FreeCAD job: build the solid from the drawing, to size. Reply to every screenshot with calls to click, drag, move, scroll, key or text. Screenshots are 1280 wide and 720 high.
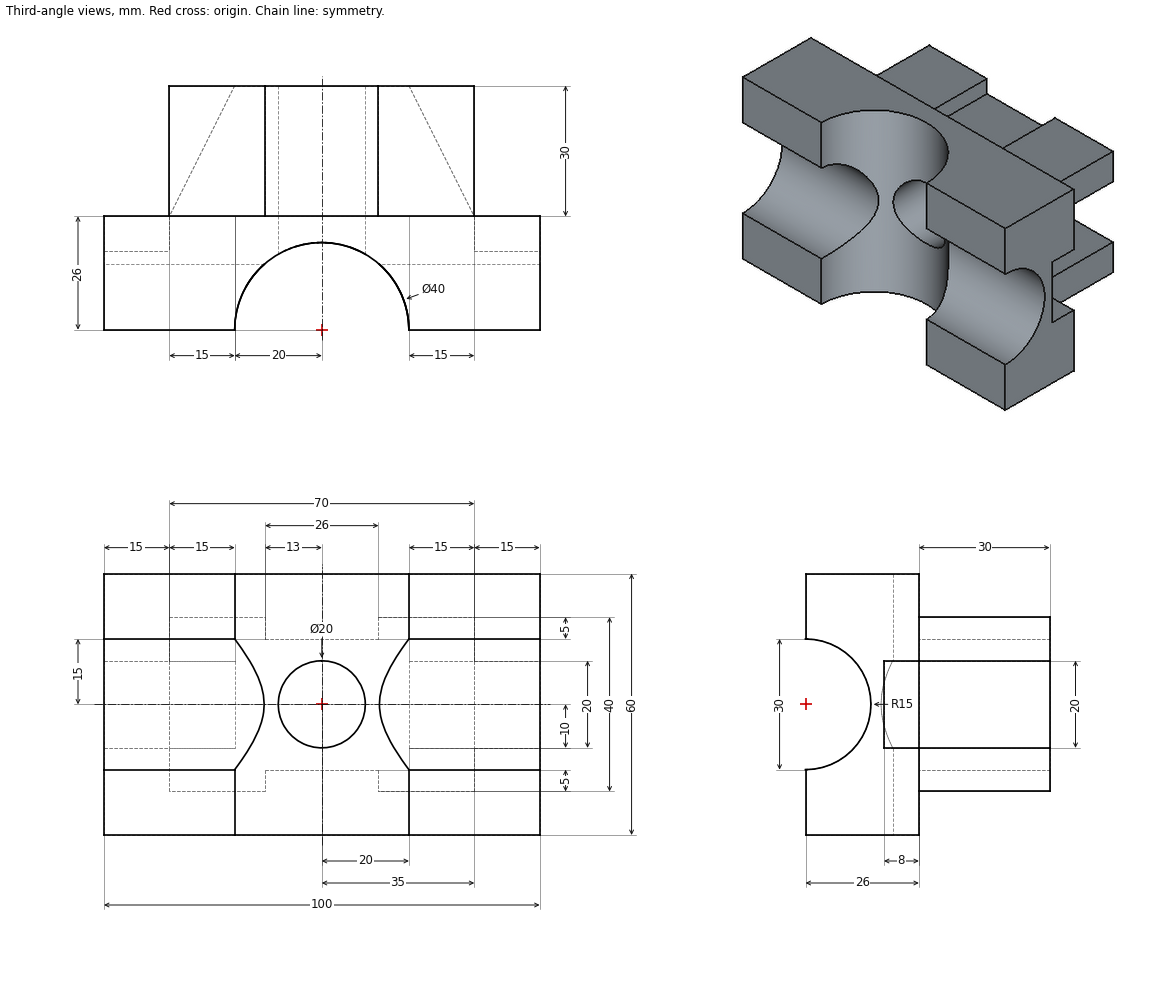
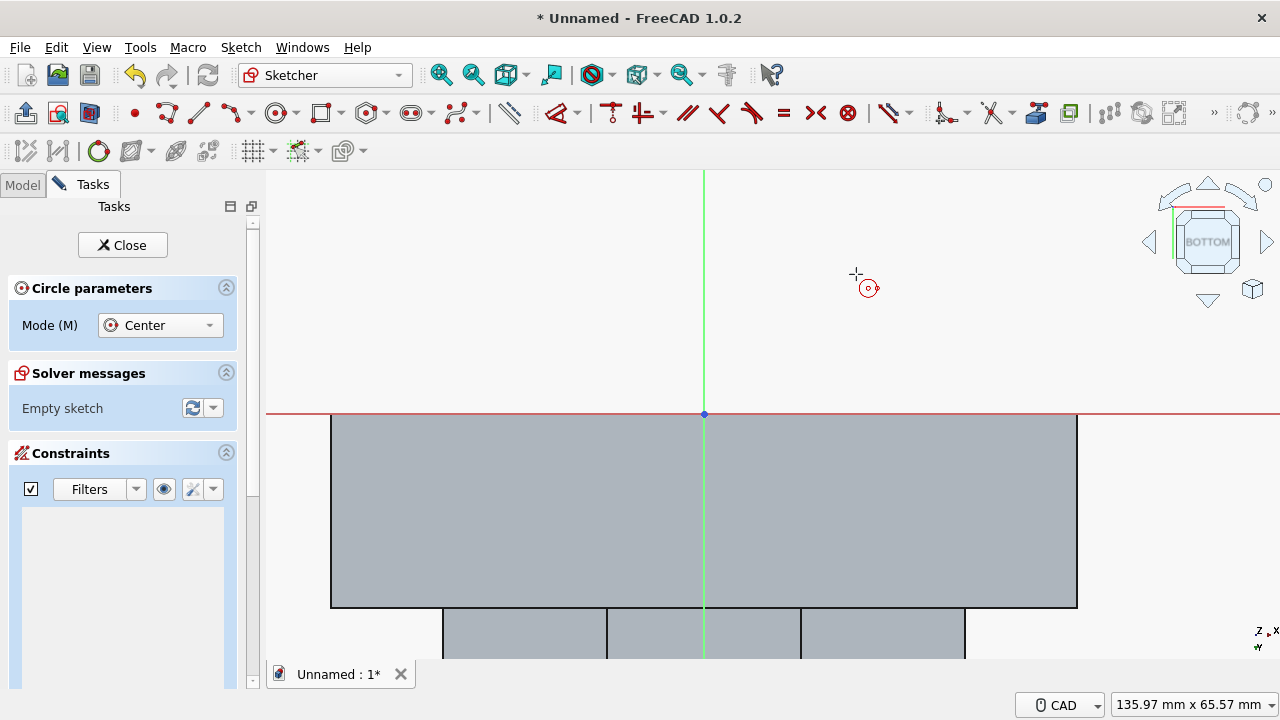
click(704, 414)
move(810, 309)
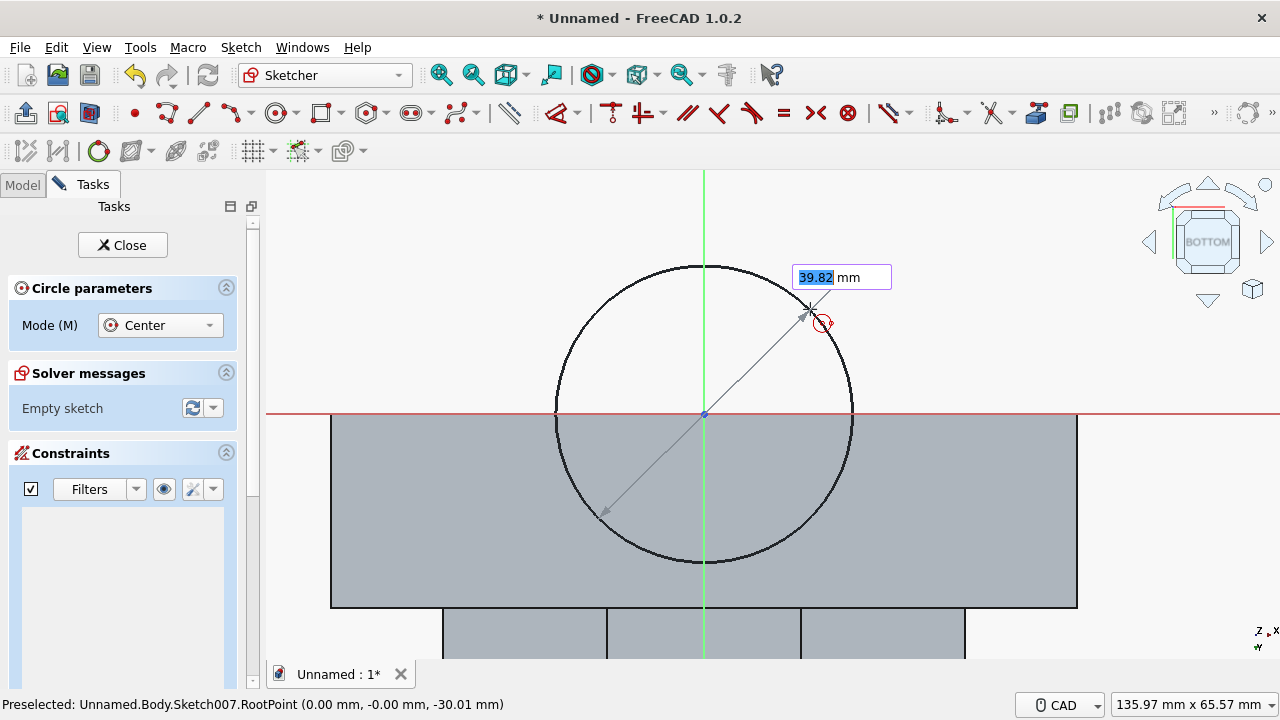
text(40)
key(Return)
key(Escape)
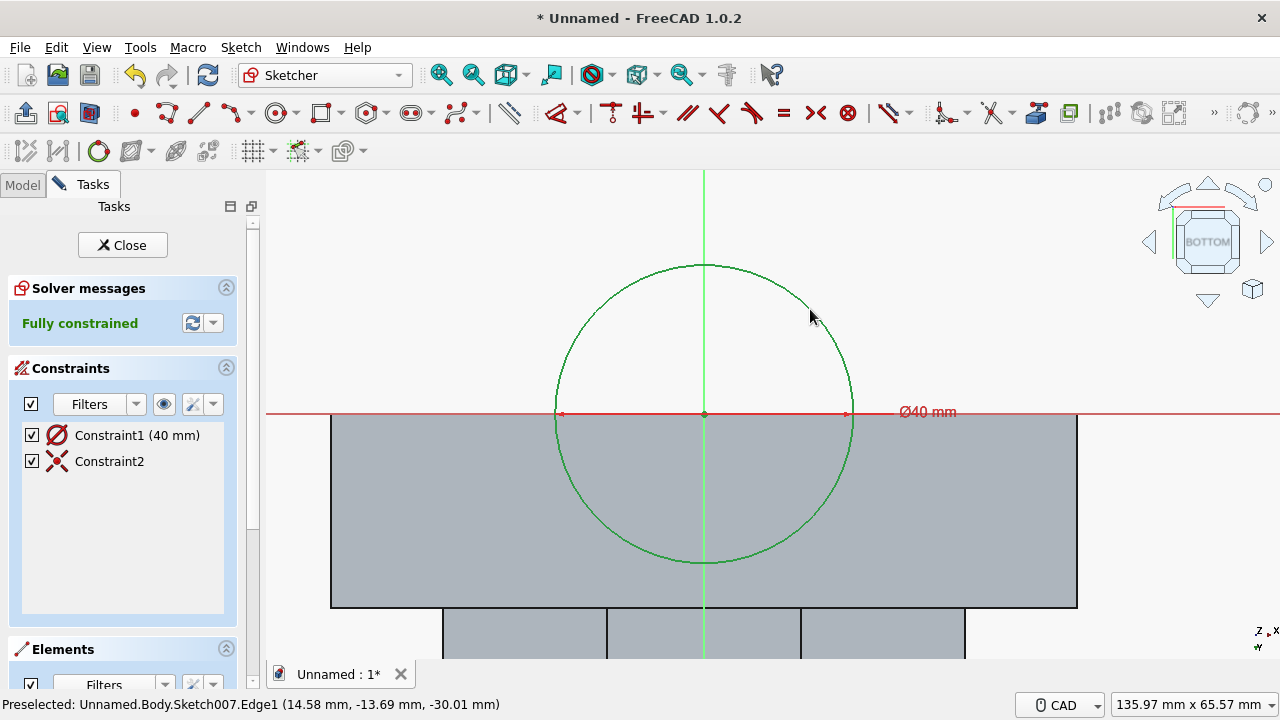
click(123, 245)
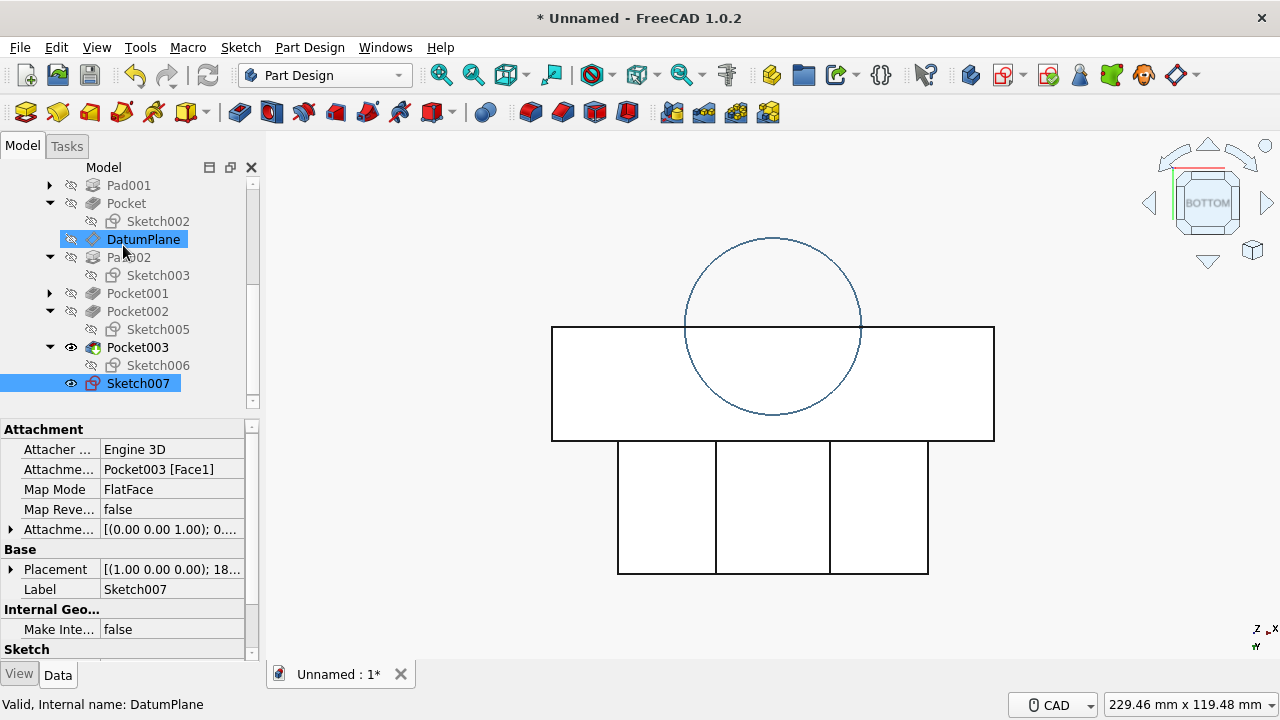
click(240, 112)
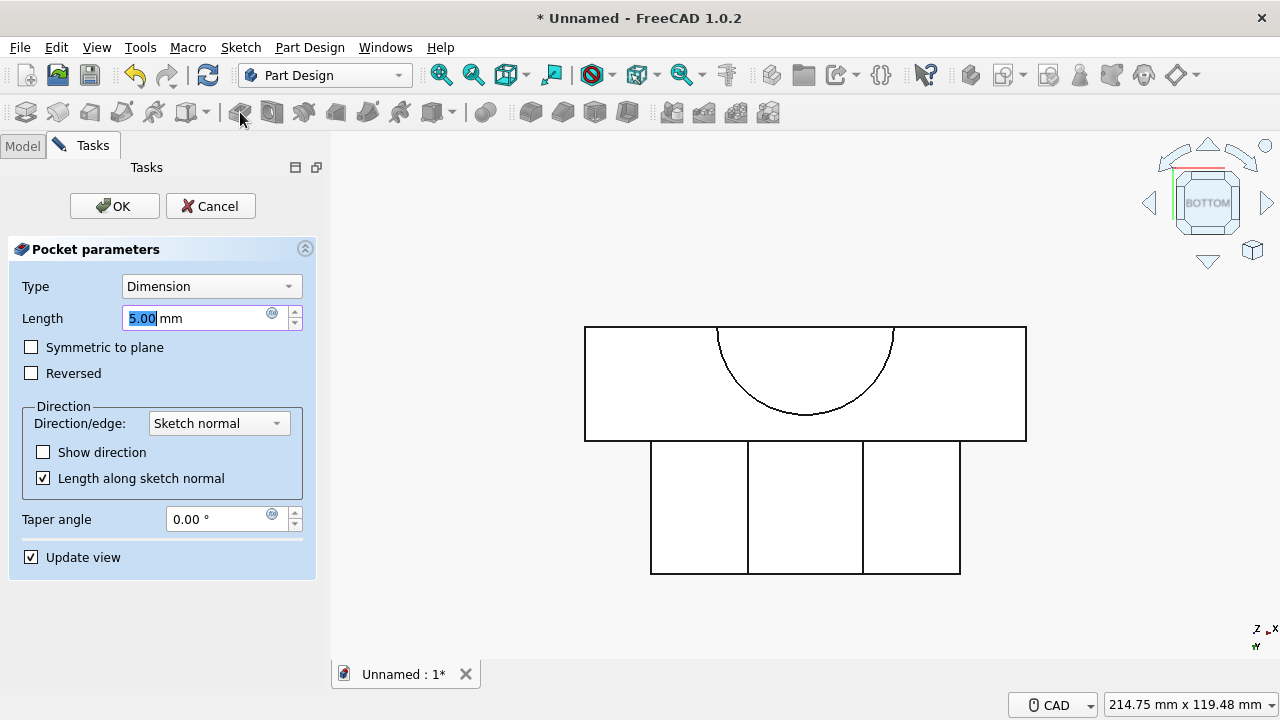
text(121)
key(Tab)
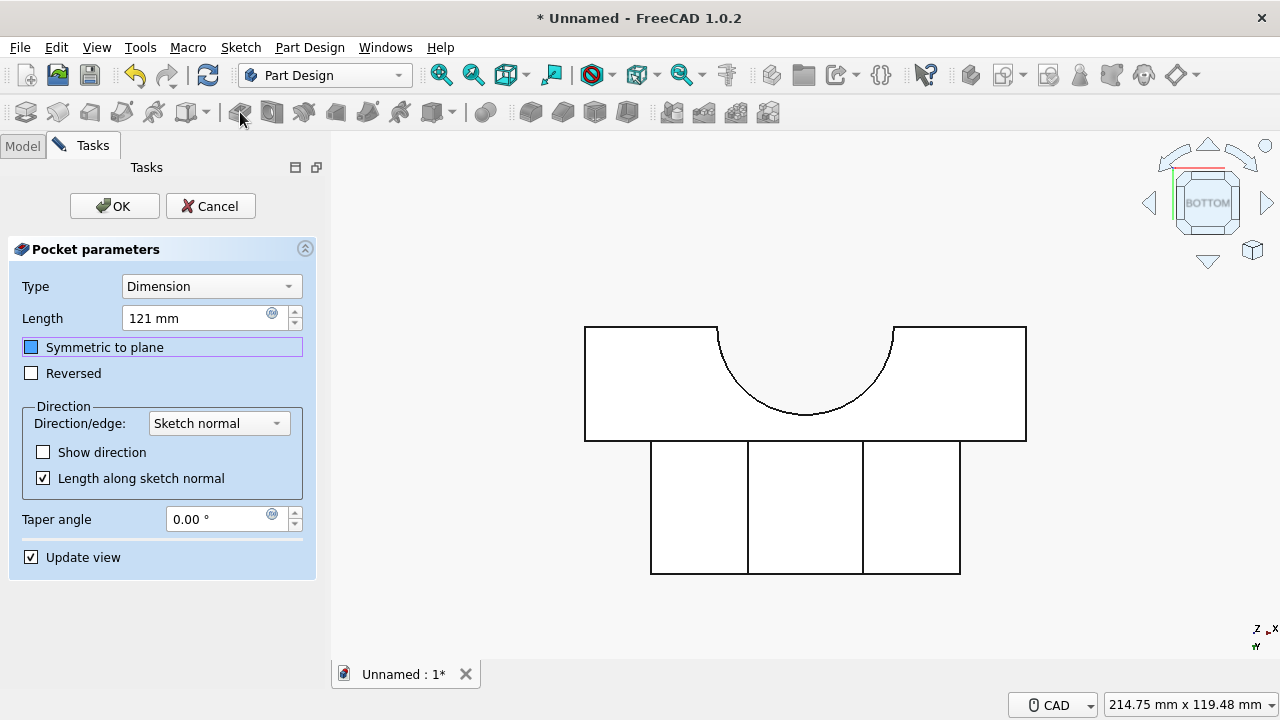
click(115, 206)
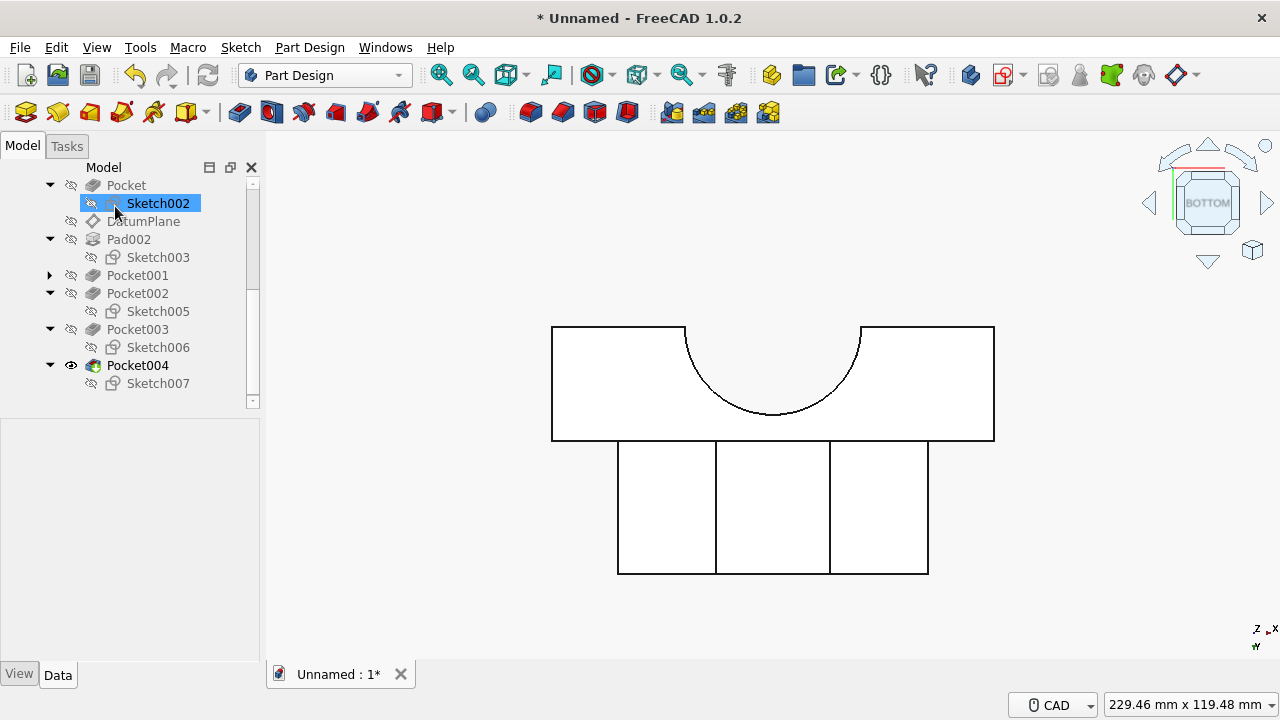
key(0)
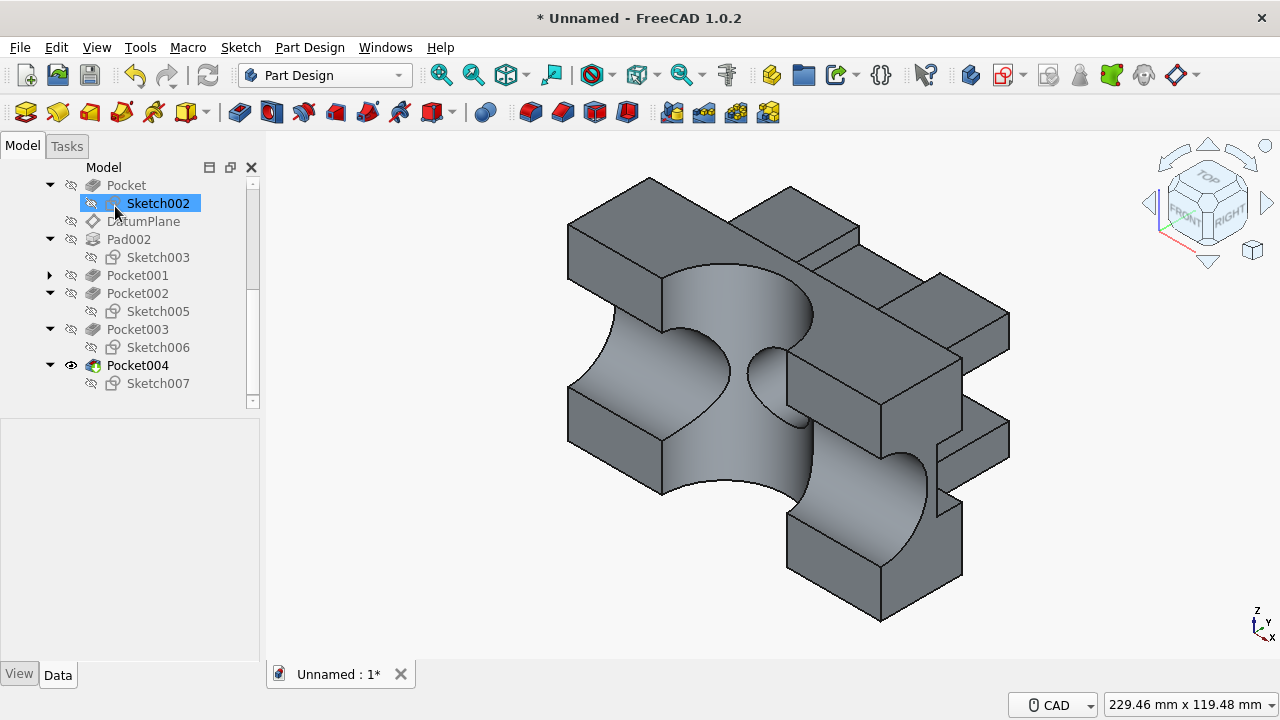
key(v)
key(f)